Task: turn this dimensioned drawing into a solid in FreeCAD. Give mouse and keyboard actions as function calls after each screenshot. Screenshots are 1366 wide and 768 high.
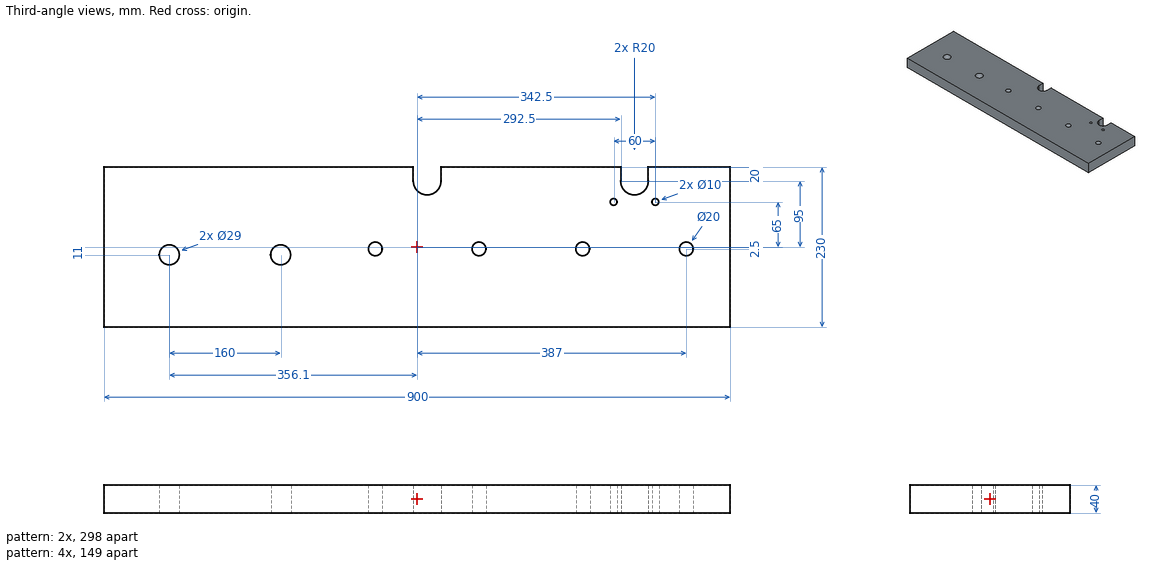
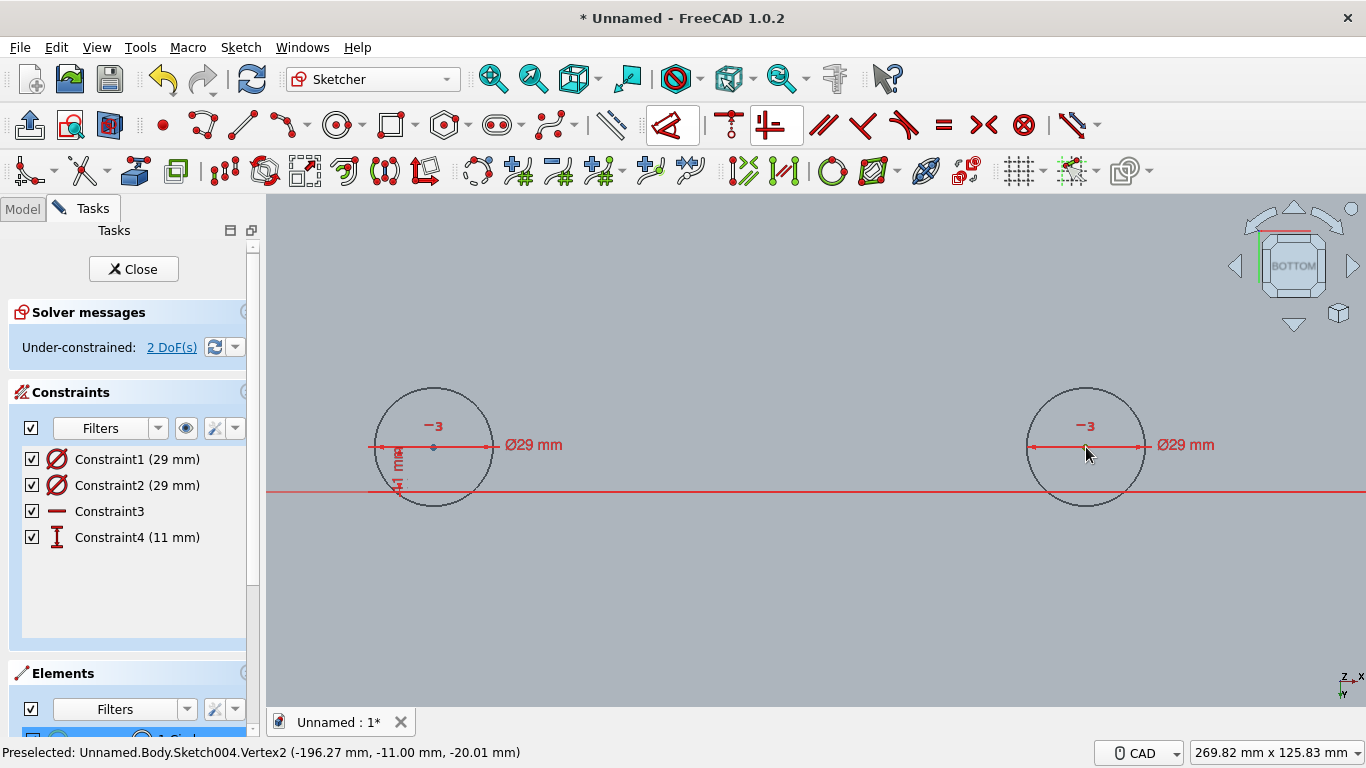
key(l)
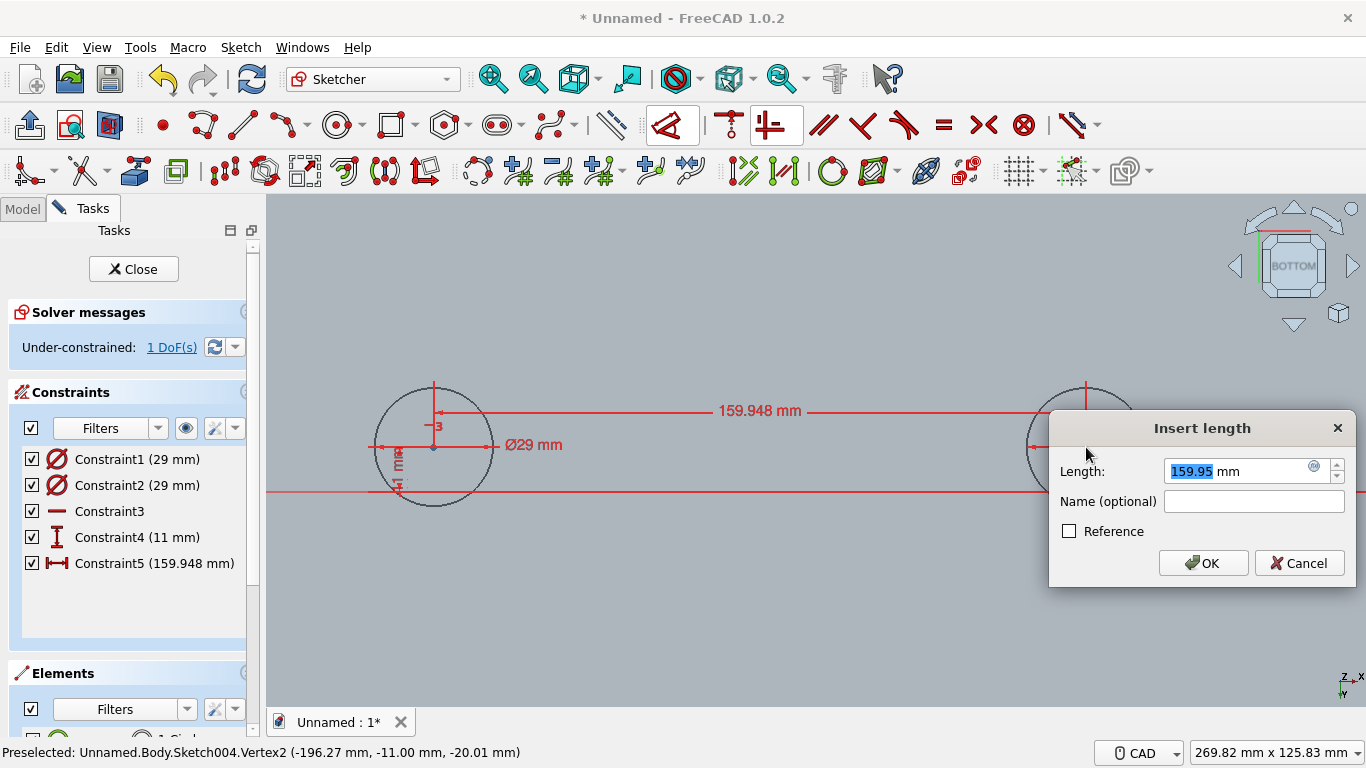
text(160)
key(Return)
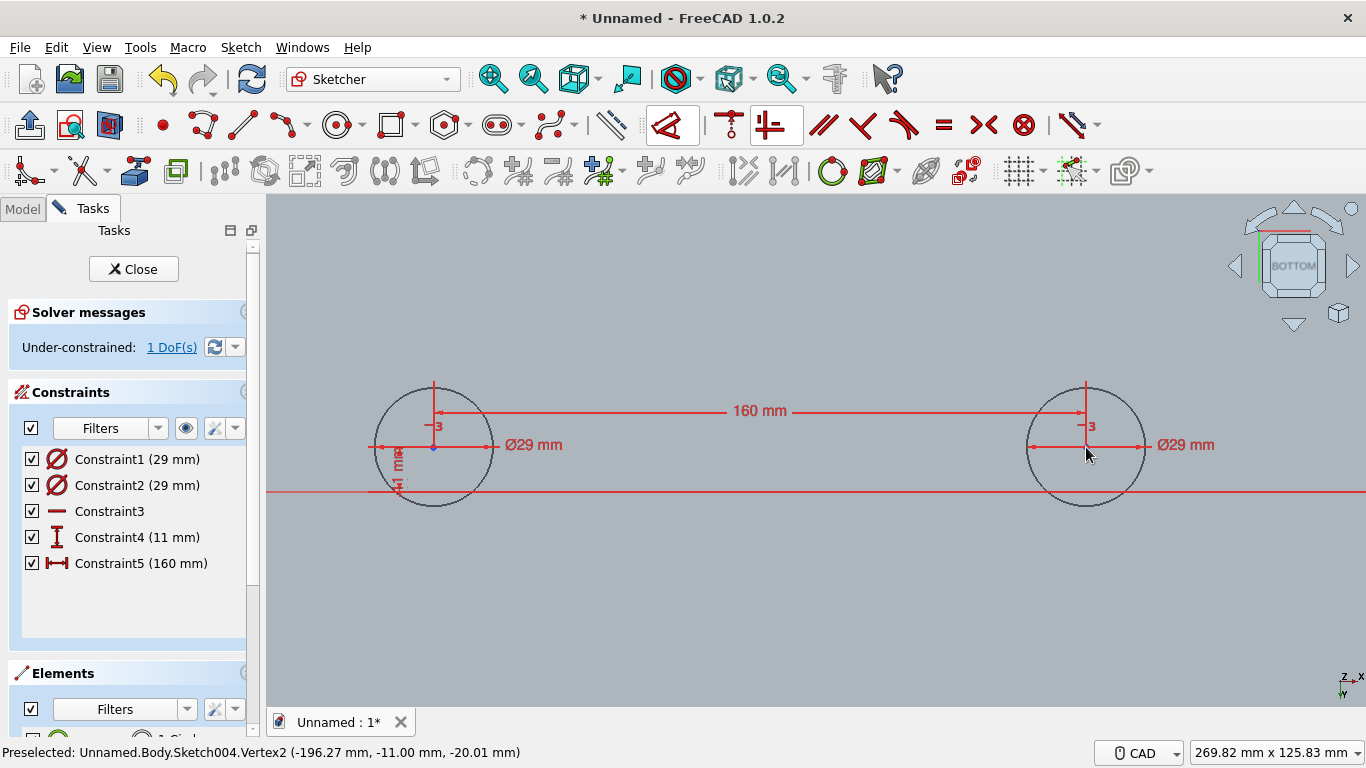
click(434, 447)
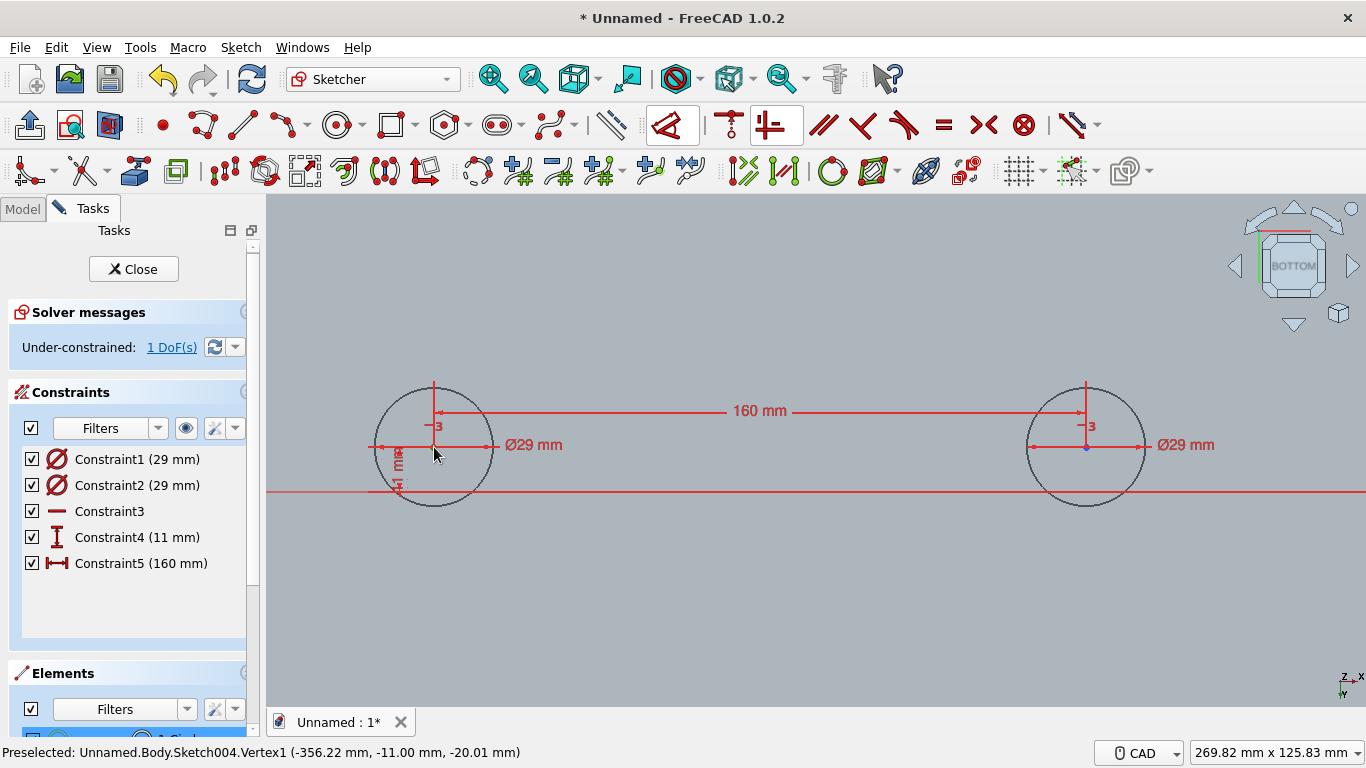
key(l)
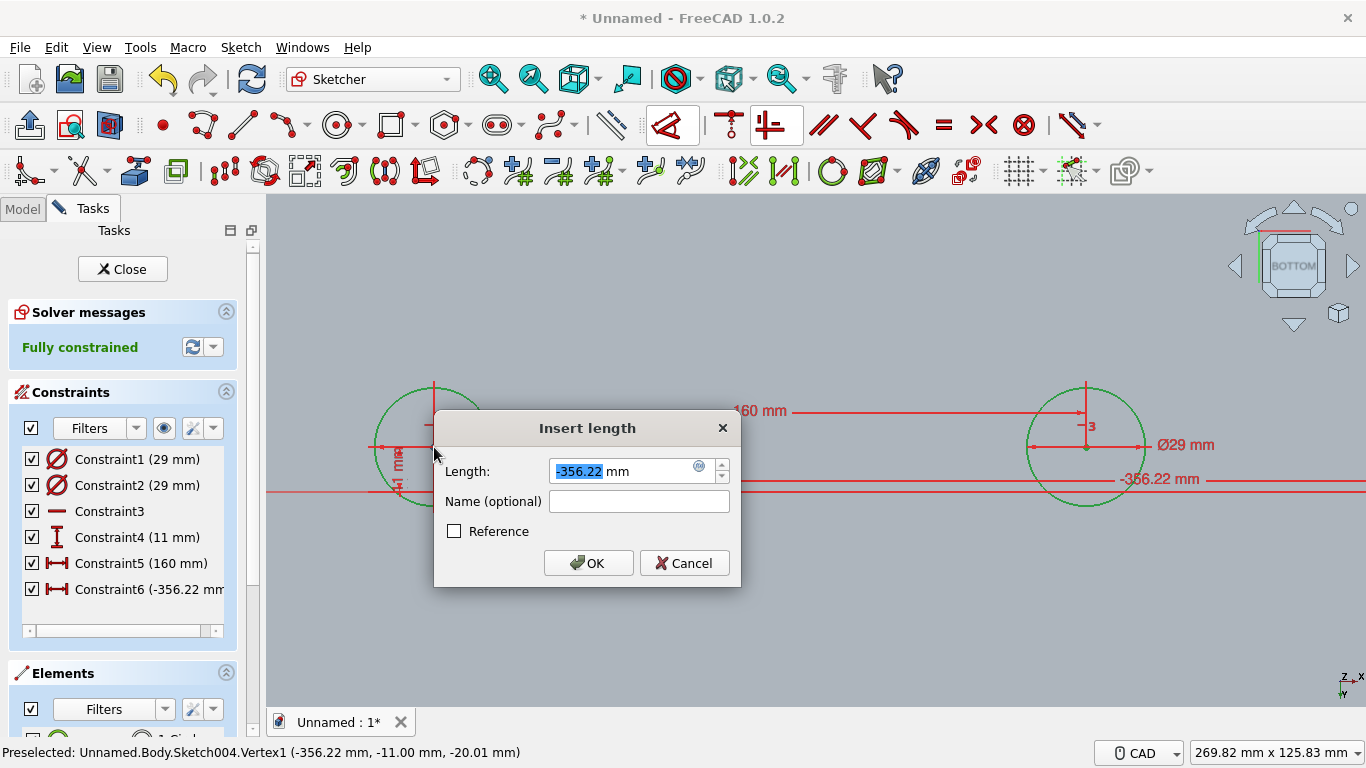
text(-356.1)
key(Return)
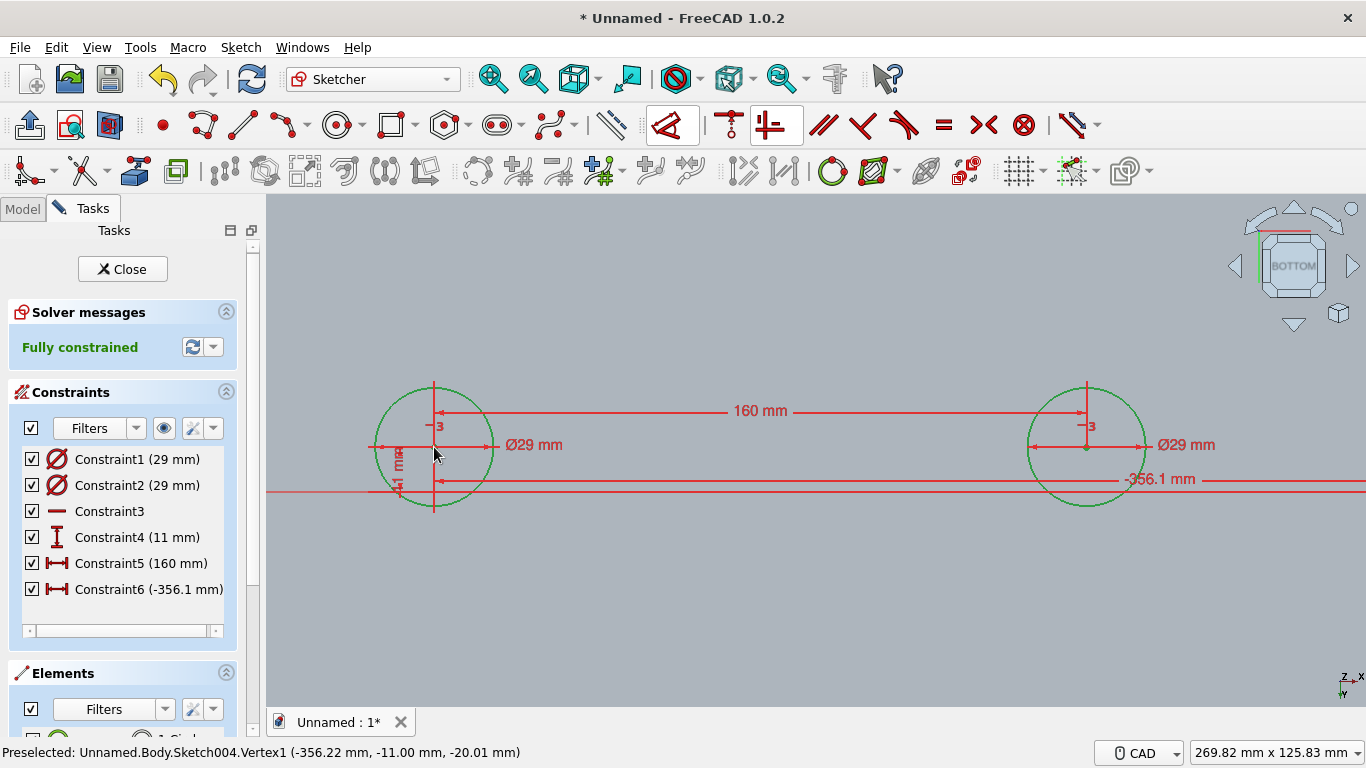
click(123, 269)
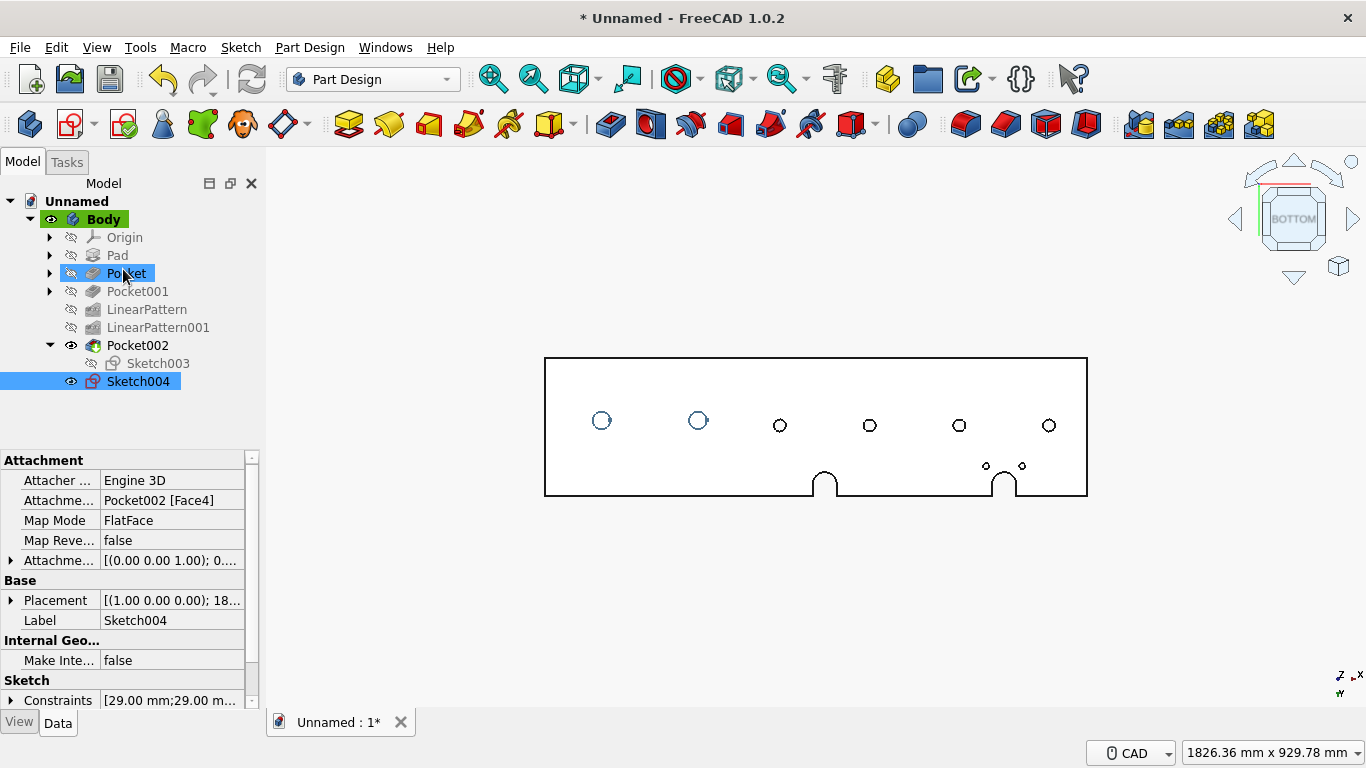
click(612, 124)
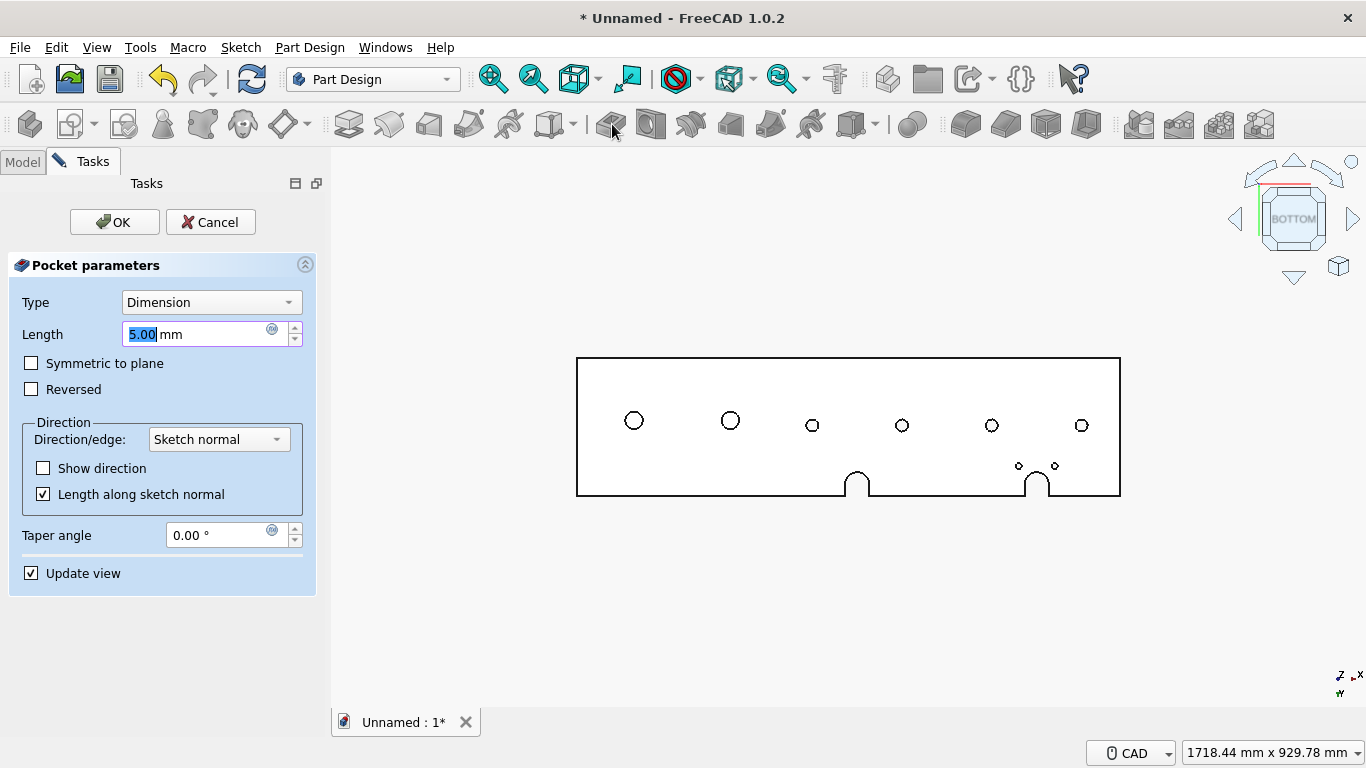
click(212, 302)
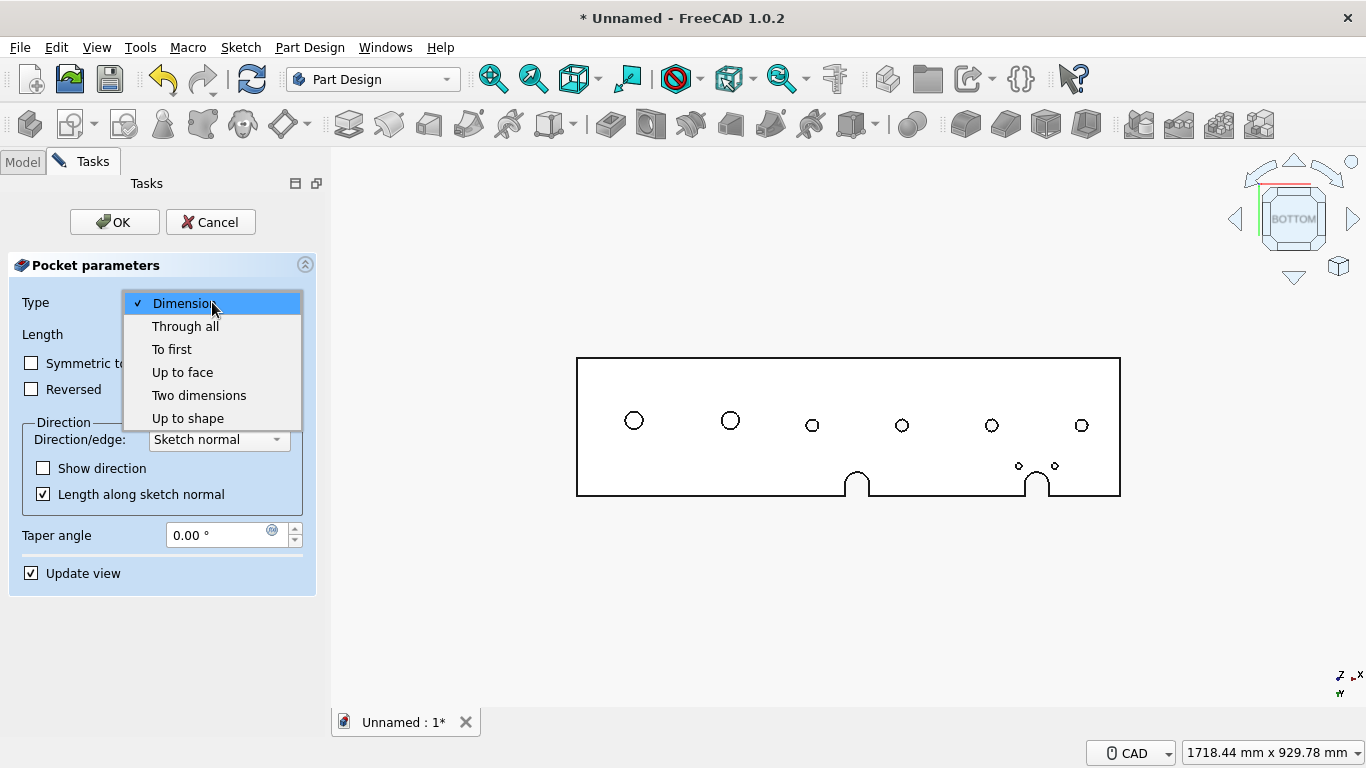
click(212, 326)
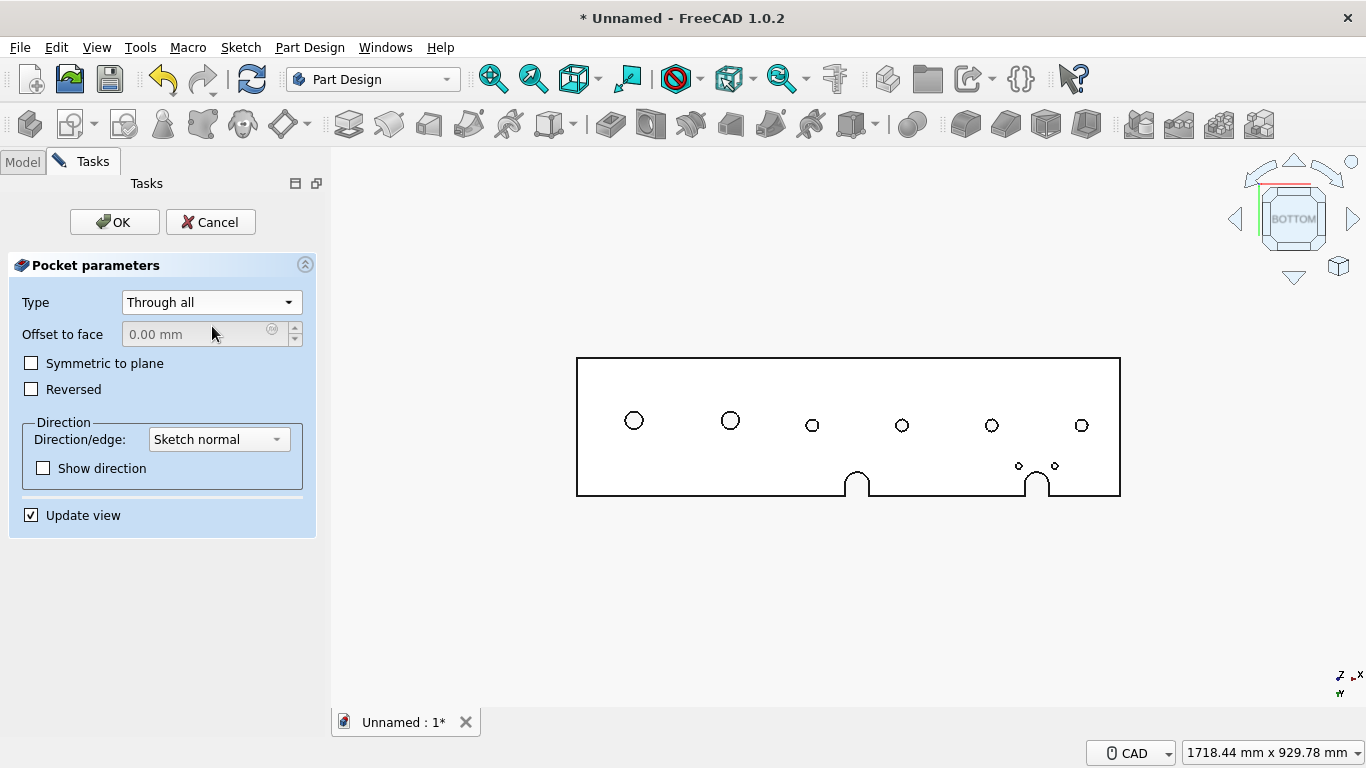
click(115, 222)